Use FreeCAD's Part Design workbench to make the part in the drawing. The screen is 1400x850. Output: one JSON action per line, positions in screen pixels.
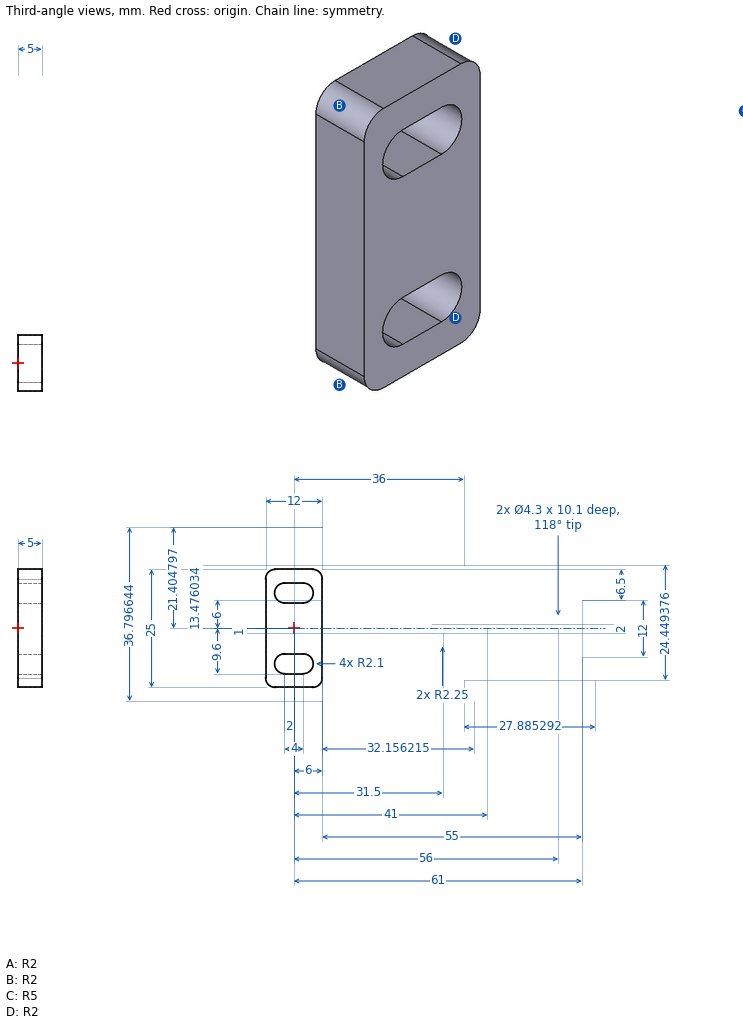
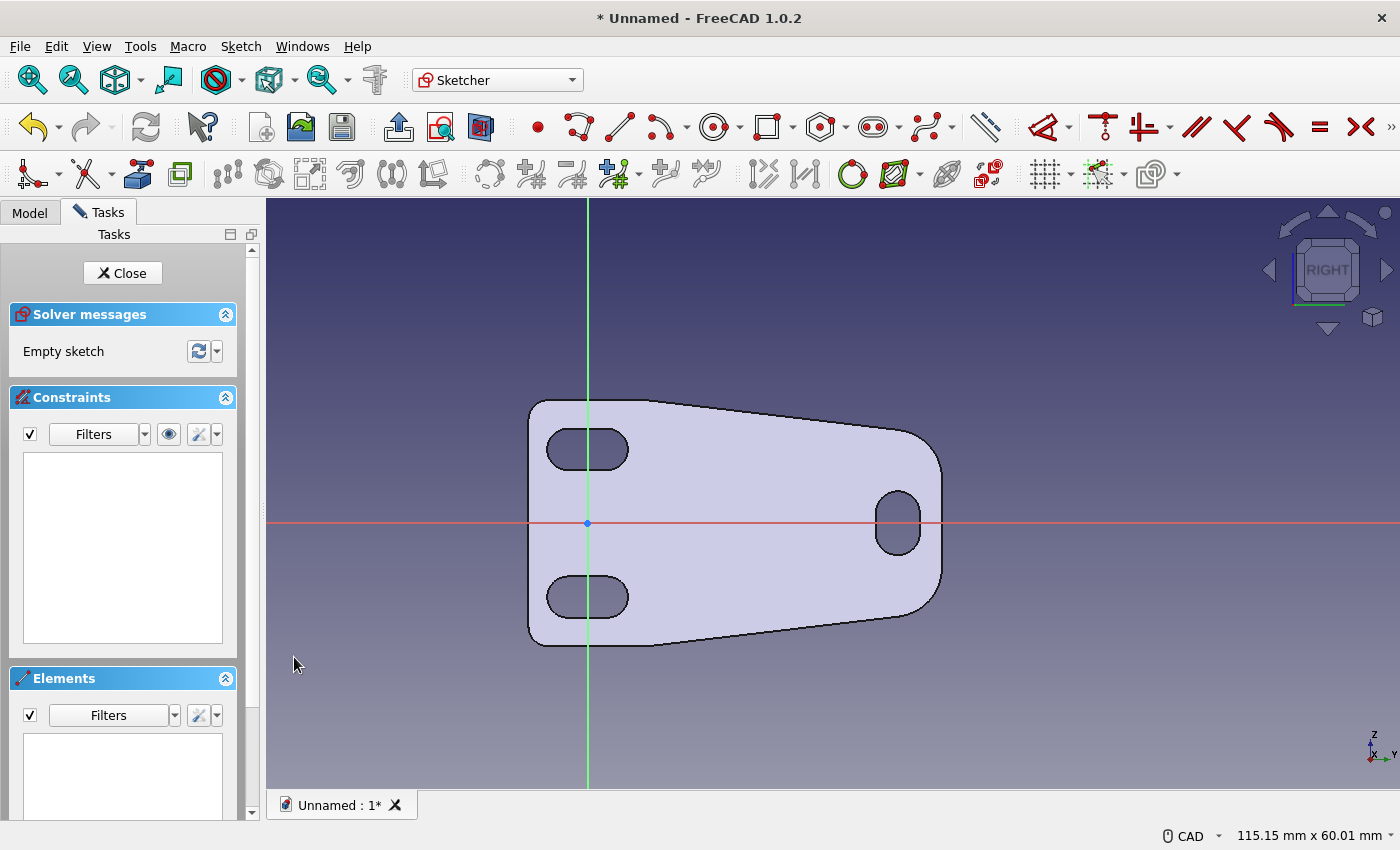
{"action": "left_click", "coordinate": [766, 128]}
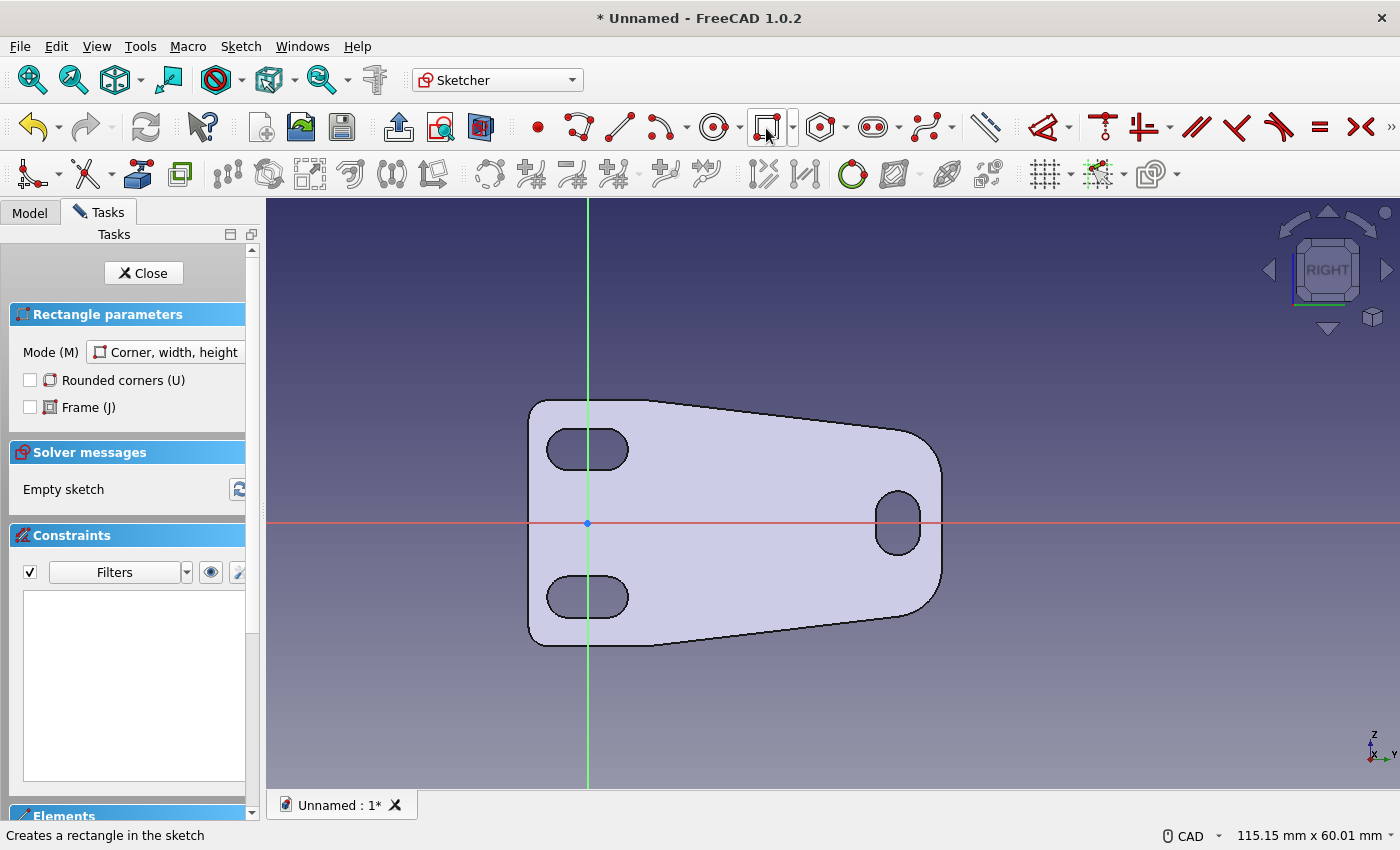
{"action": "left_click", "coordinate": [647, 312]}
{"action": "left_click", "coordinate": [963, 675]}
{"action": "key", "text": "Escape"}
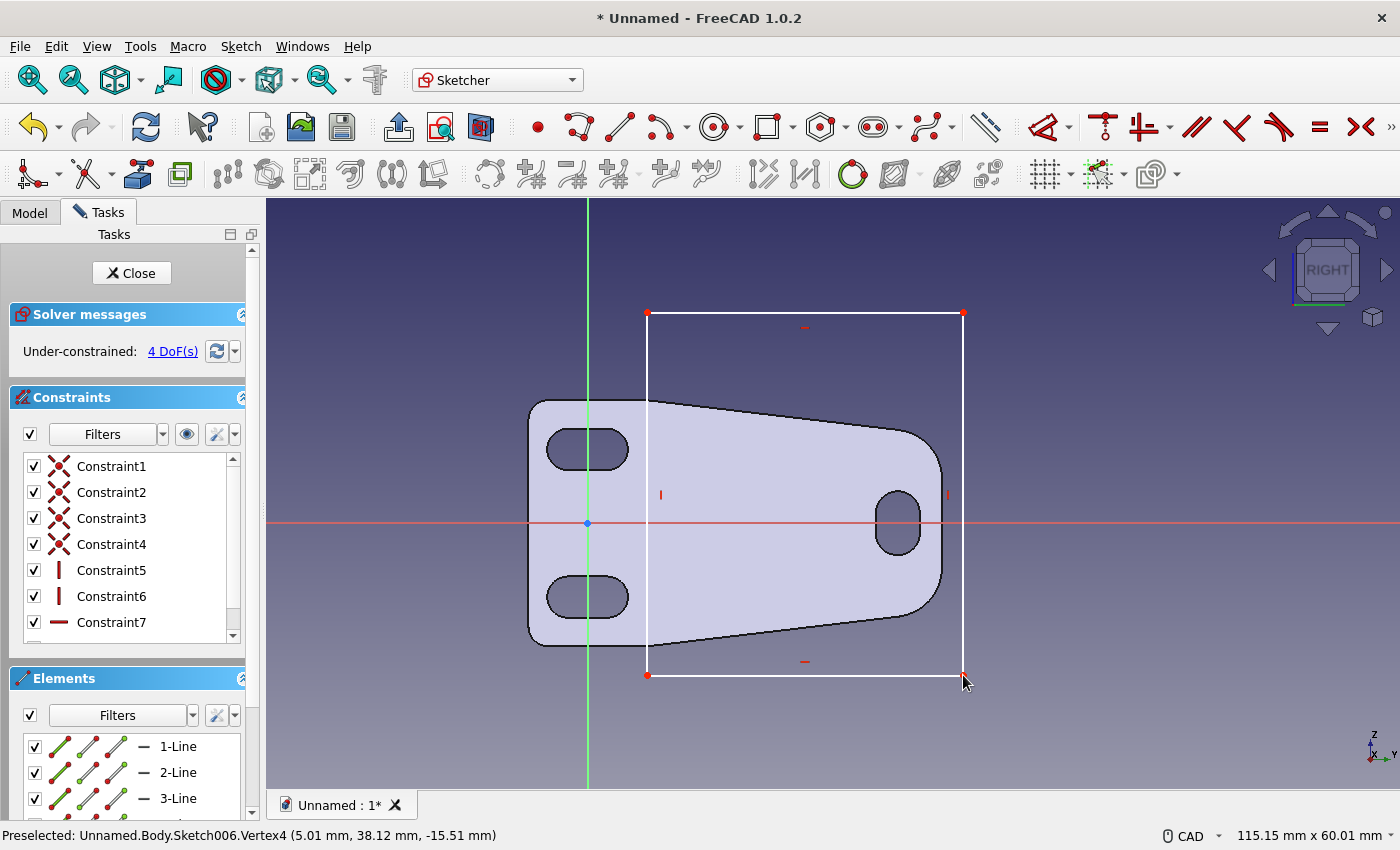
{"action": "key", "text": "d"}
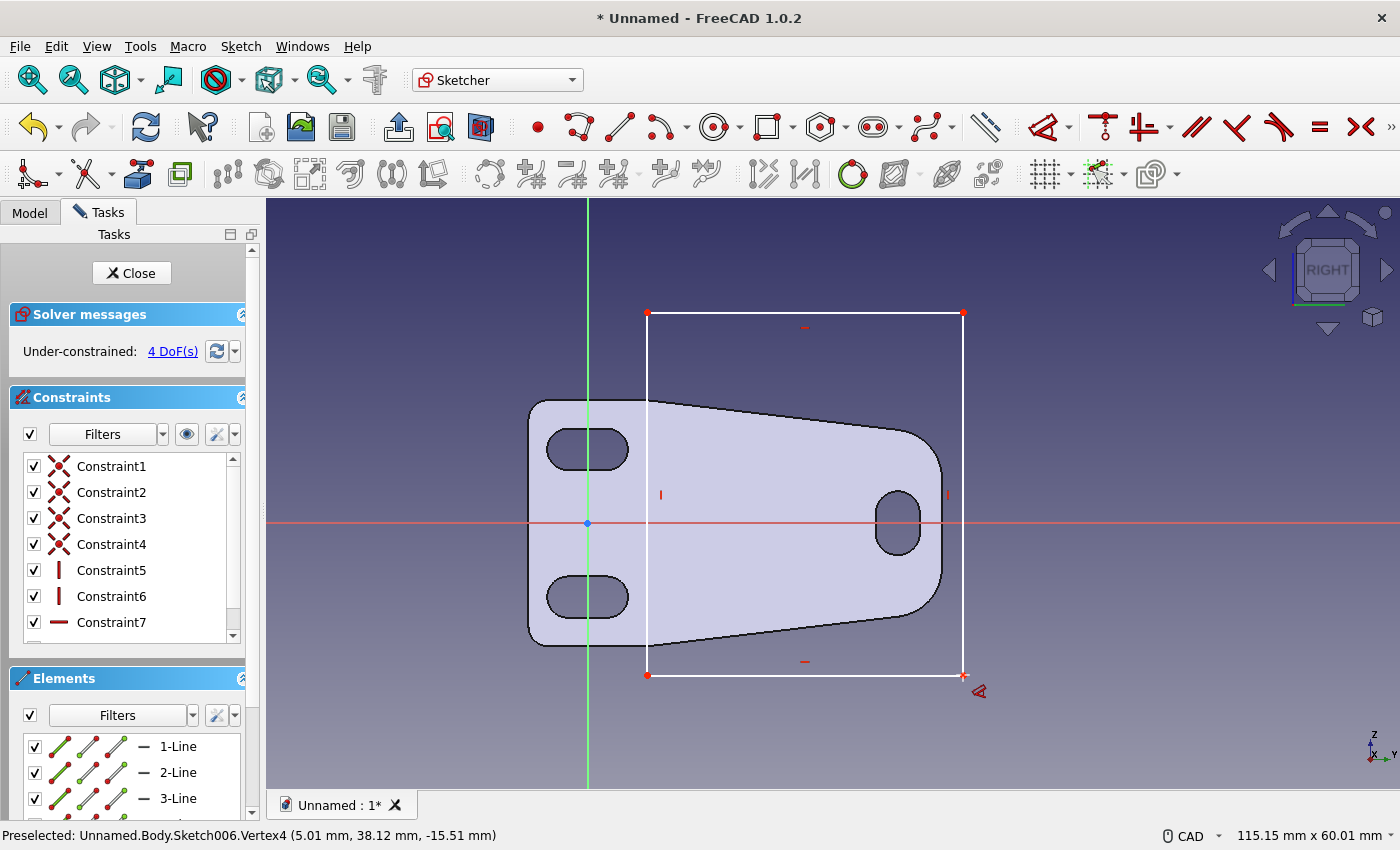
{"action": "left_click", "coordinate": [647, 313]}
{"action": "left_click", "coordinate": [617, 279]}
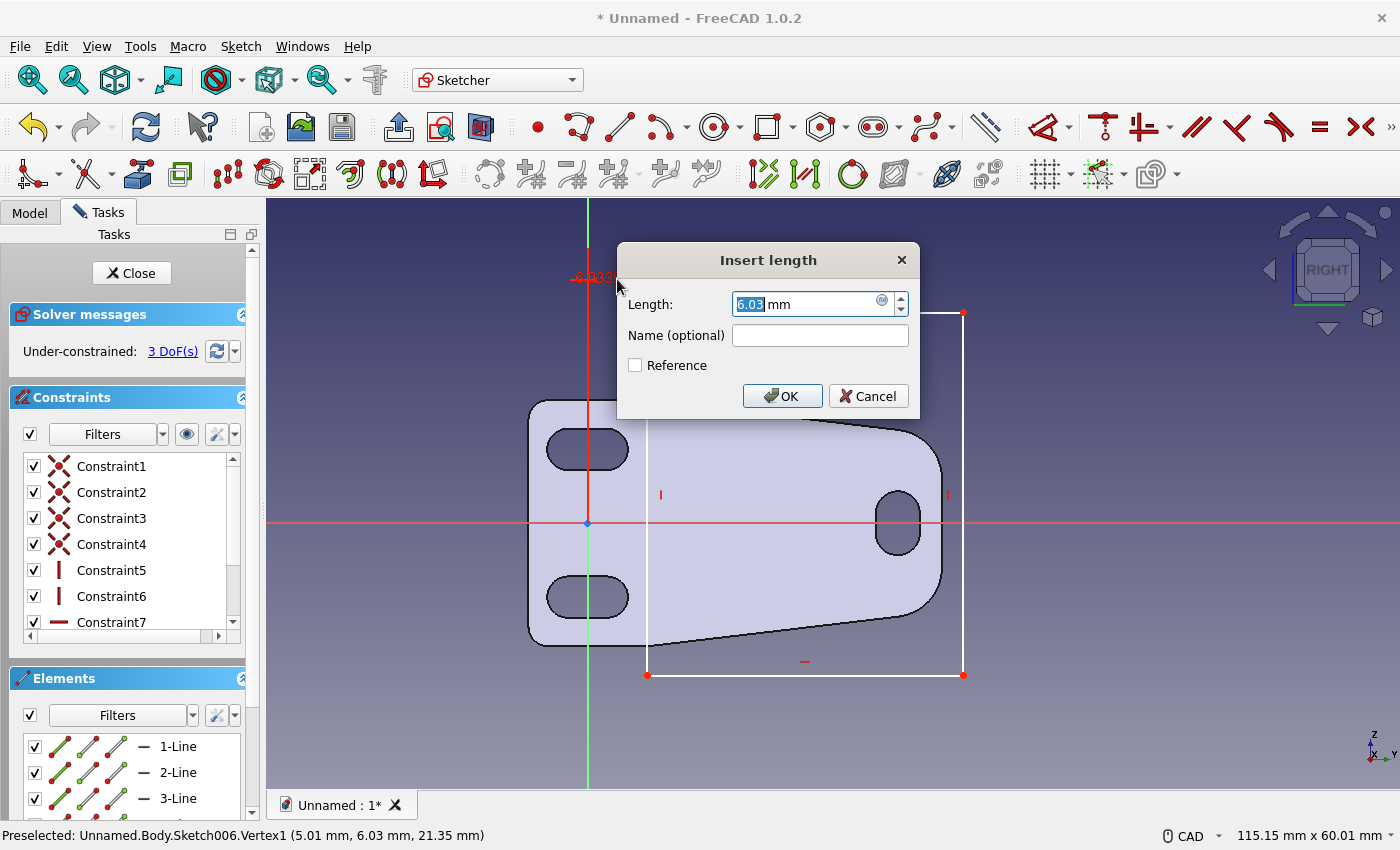
{"action": "type", "text": "6"}
{"action": "key", "text": "Return"}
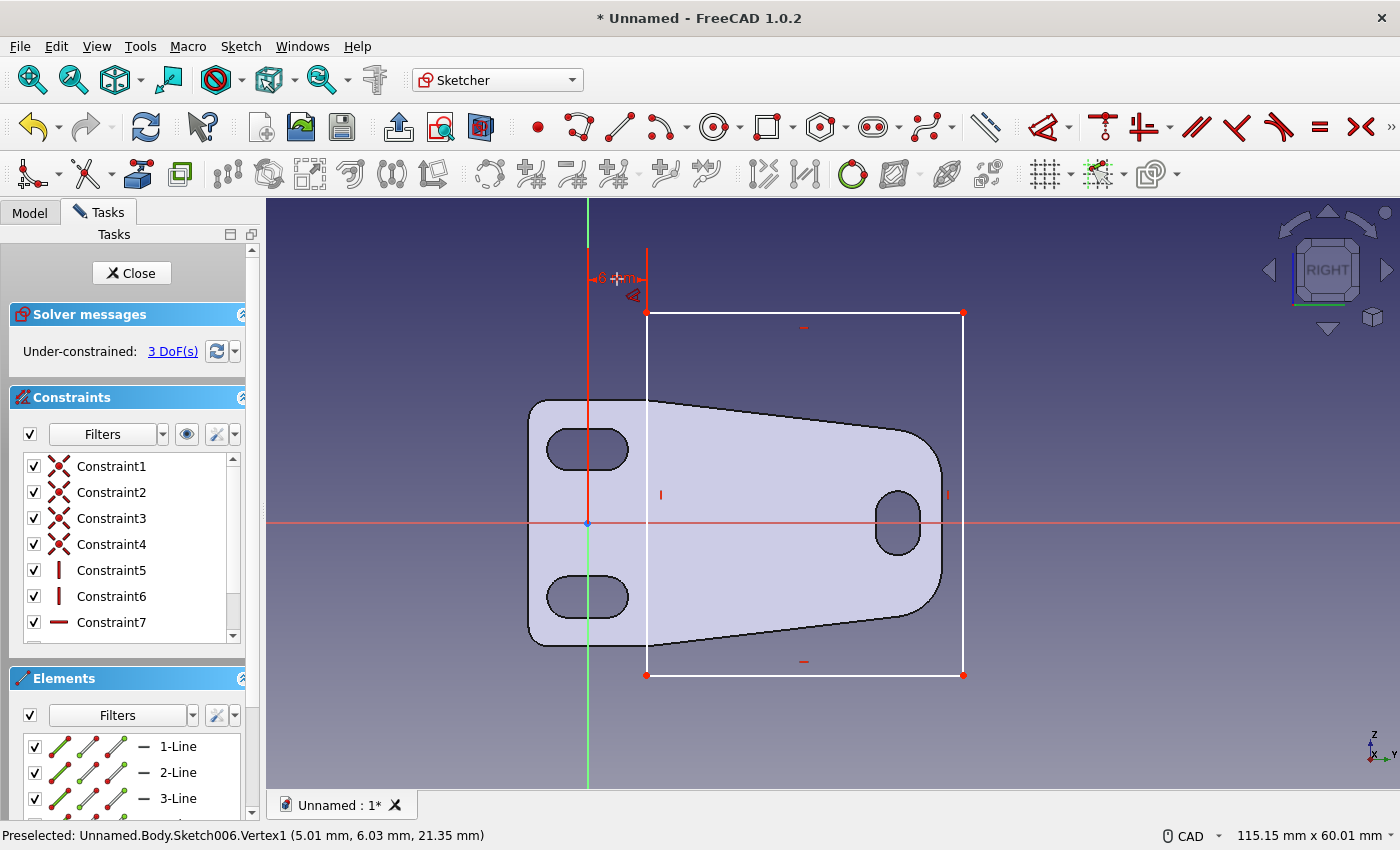
{"action": "left_click", "coordinate": [647, 422]}
{"action": "left_click", "coordinate": [613, 495]}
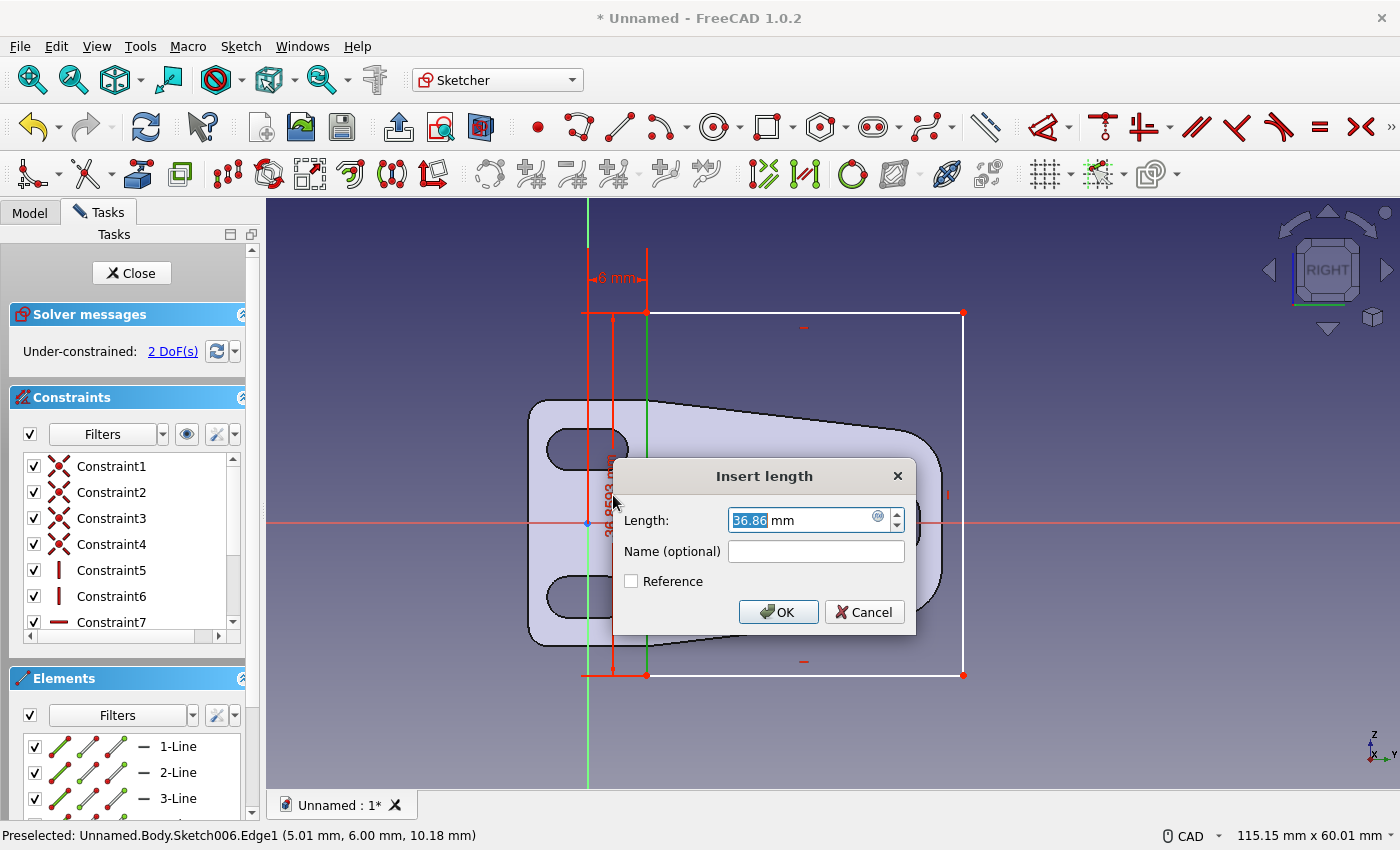
{"action": "type", "text": "36.796644"}
{"action": "key", "text": "Return"}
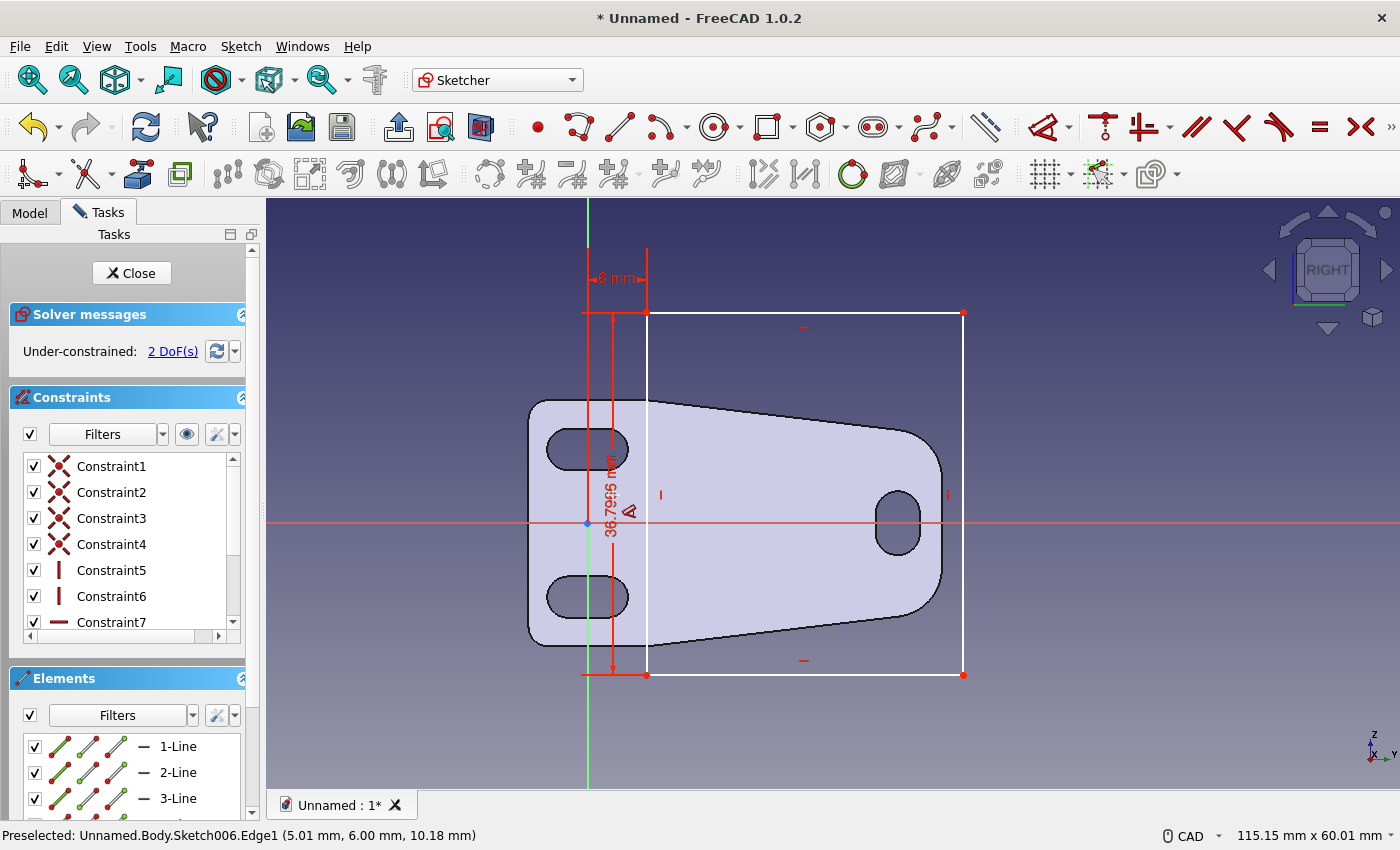
{"action": "left_click", "coordinate": [742, 675]}
{"action": "left_click", "coordinate": [805, 709]}